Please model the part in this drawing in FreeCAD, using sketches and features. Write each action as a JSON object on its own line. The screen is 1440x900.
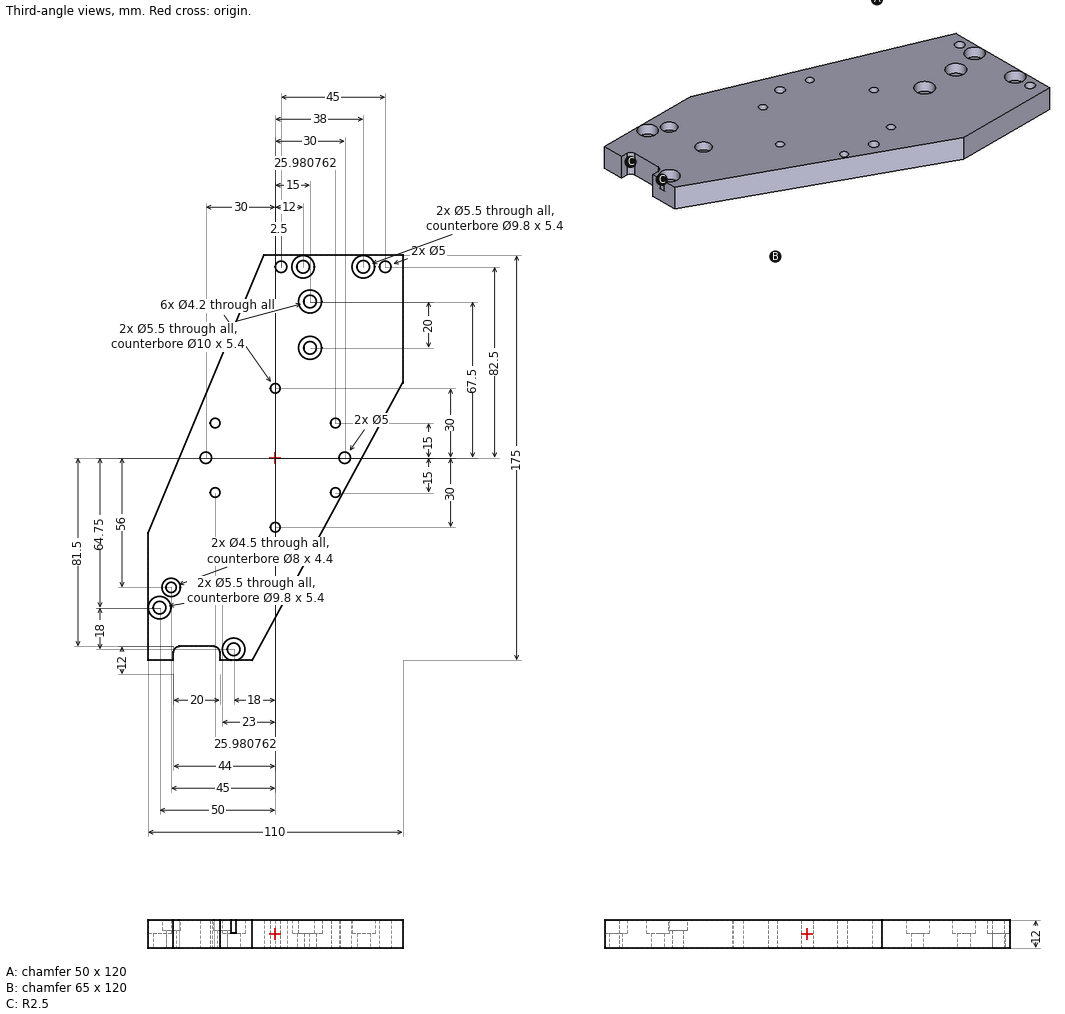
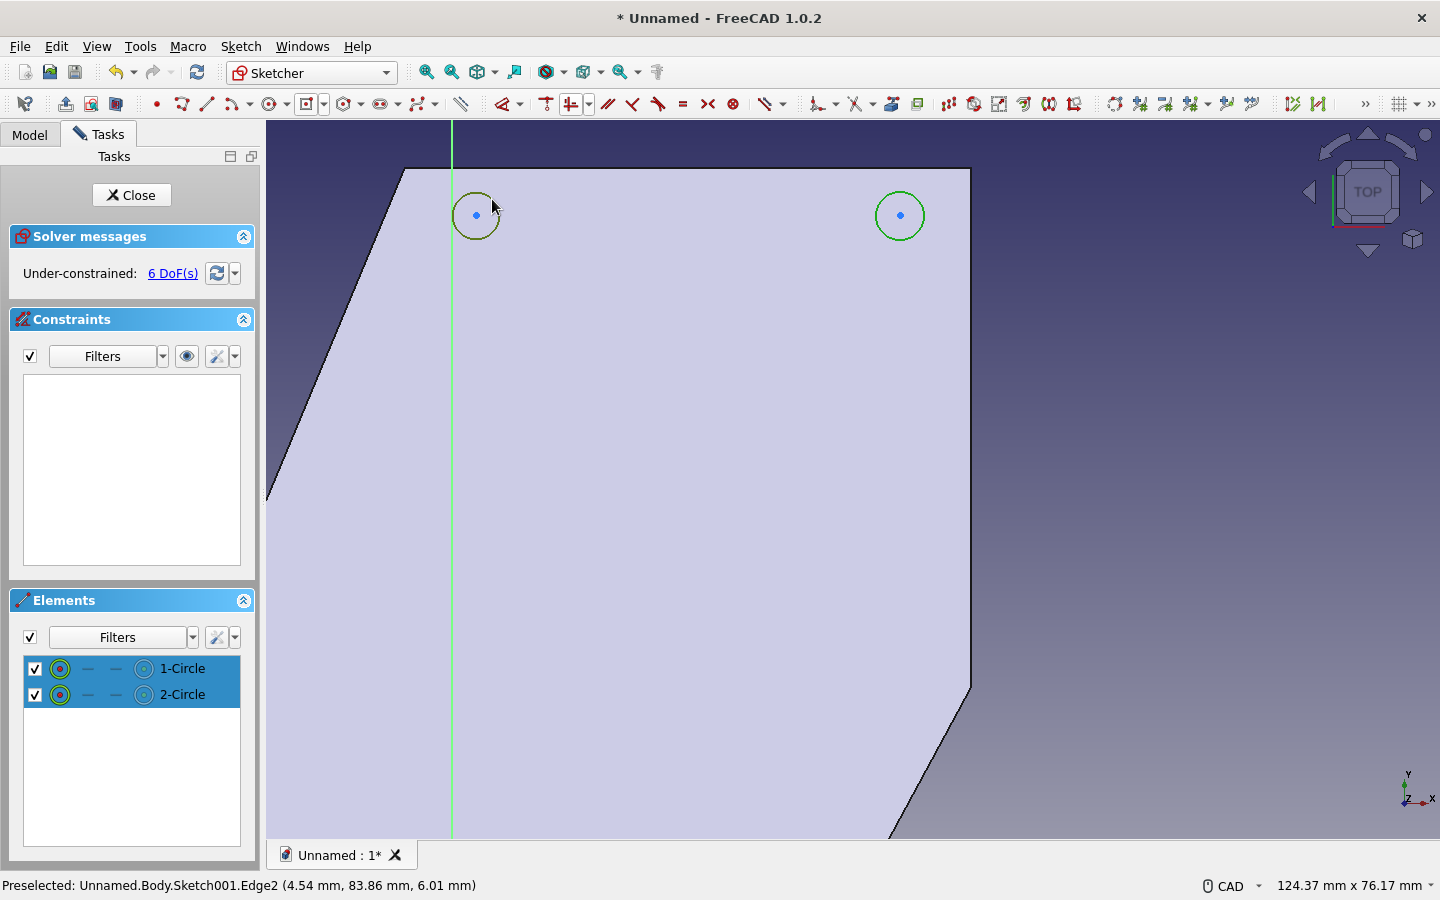
{"action": "key", "text": "e"}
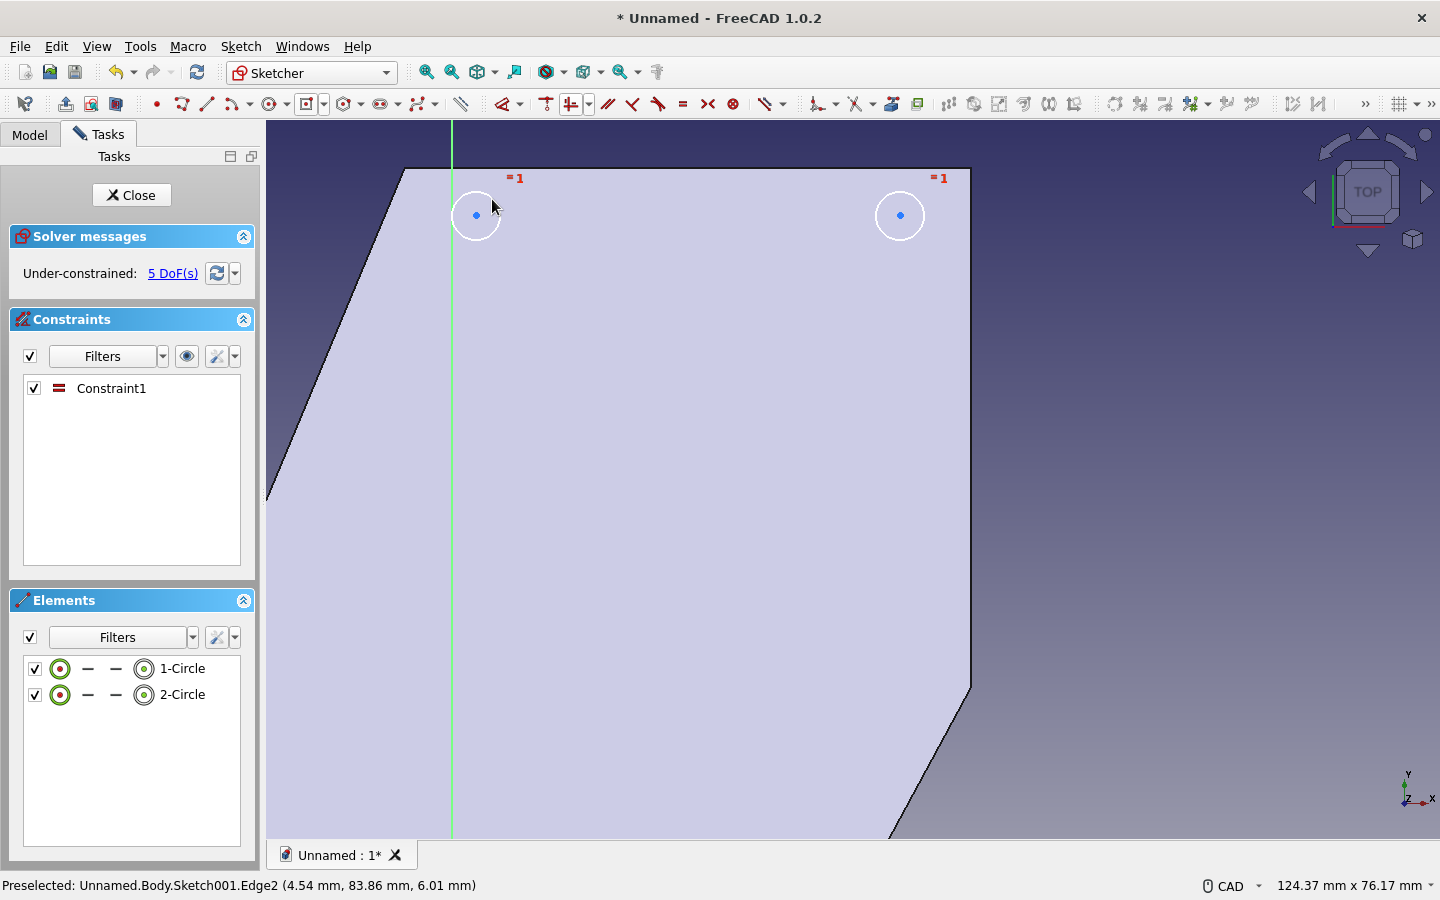
{"action": "left_click", "coordinate": [900, 216]}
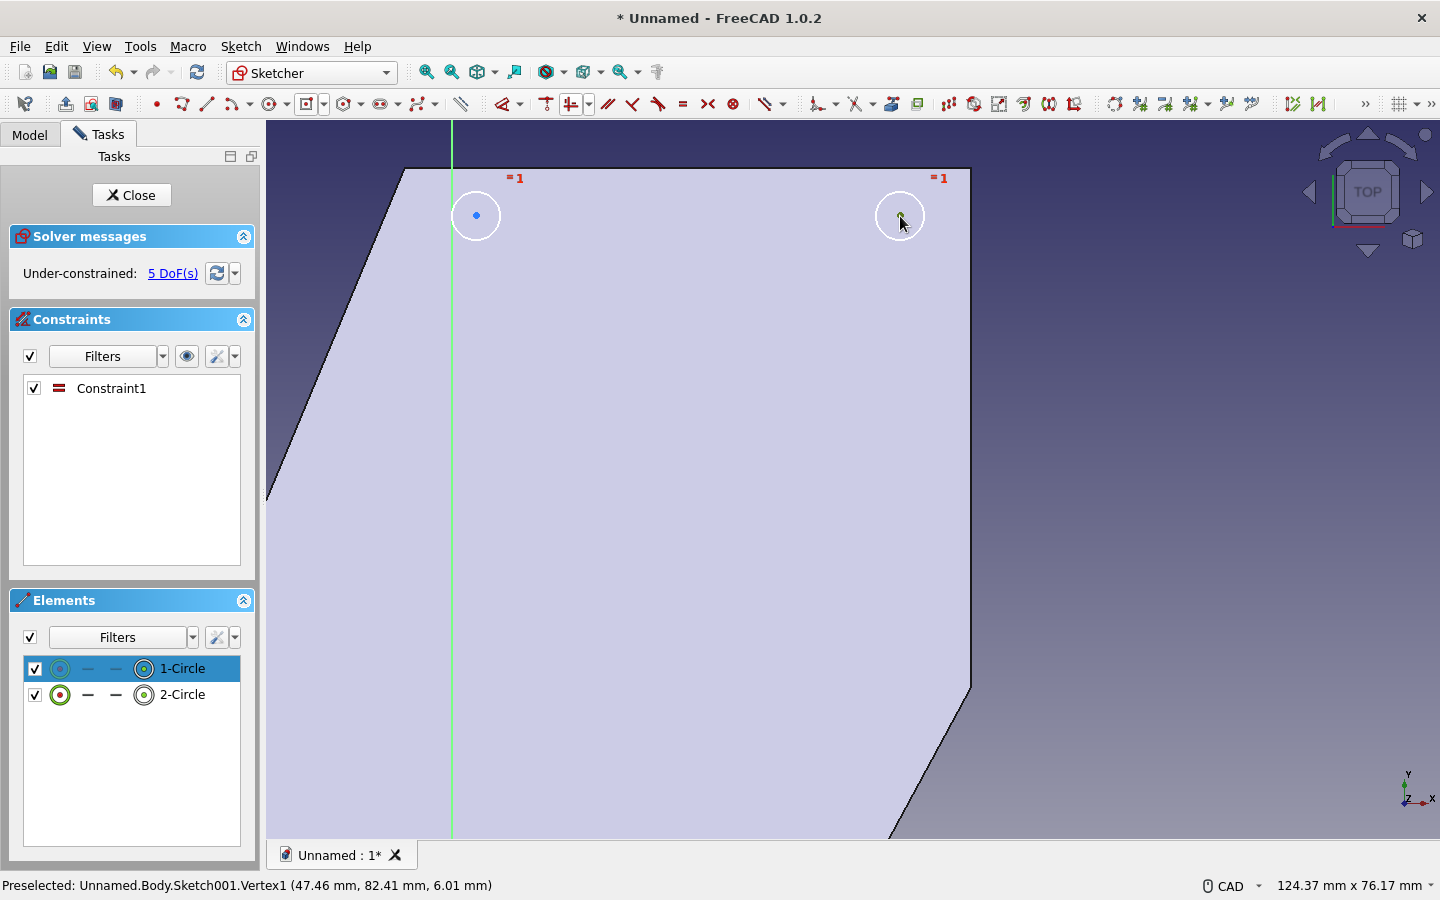
{"action": "left_click", "coordinate": [476, 216]}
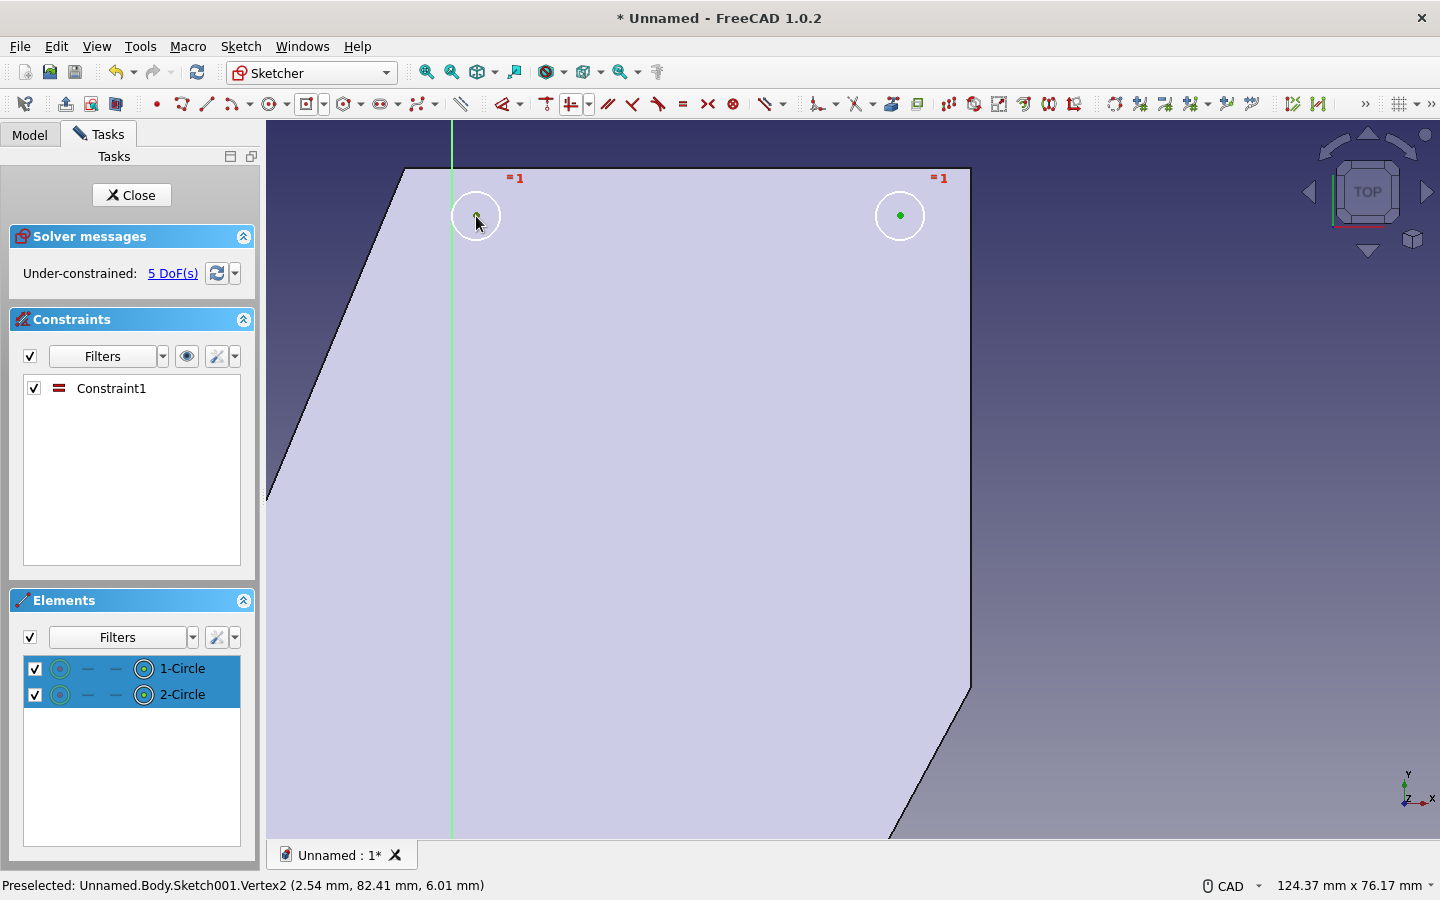
{"action": "key", "text": "h"}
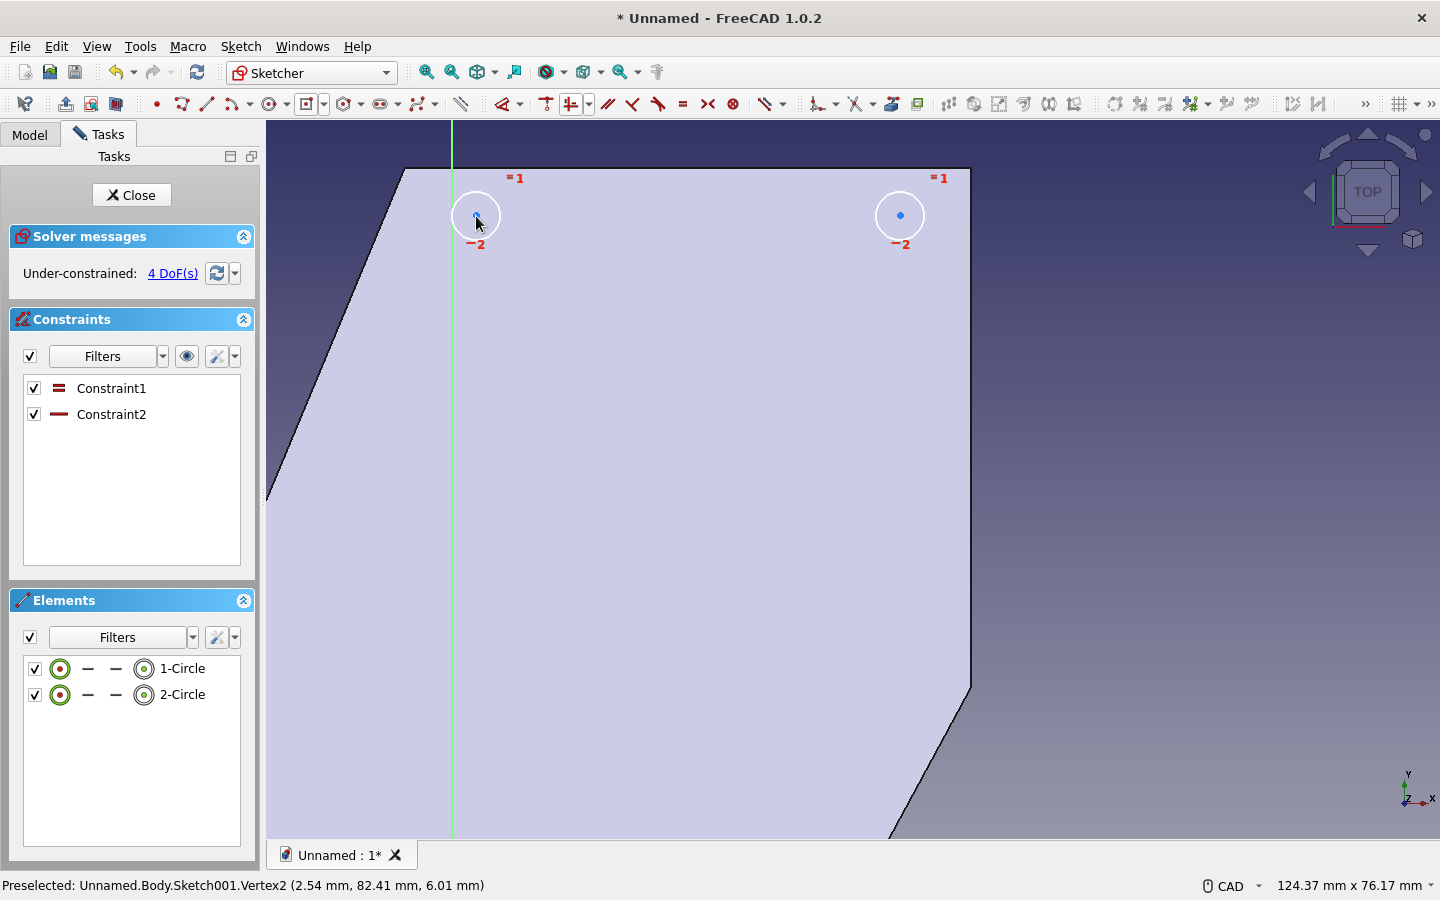
{"action": "left_click", "coordinate": [917, 199]}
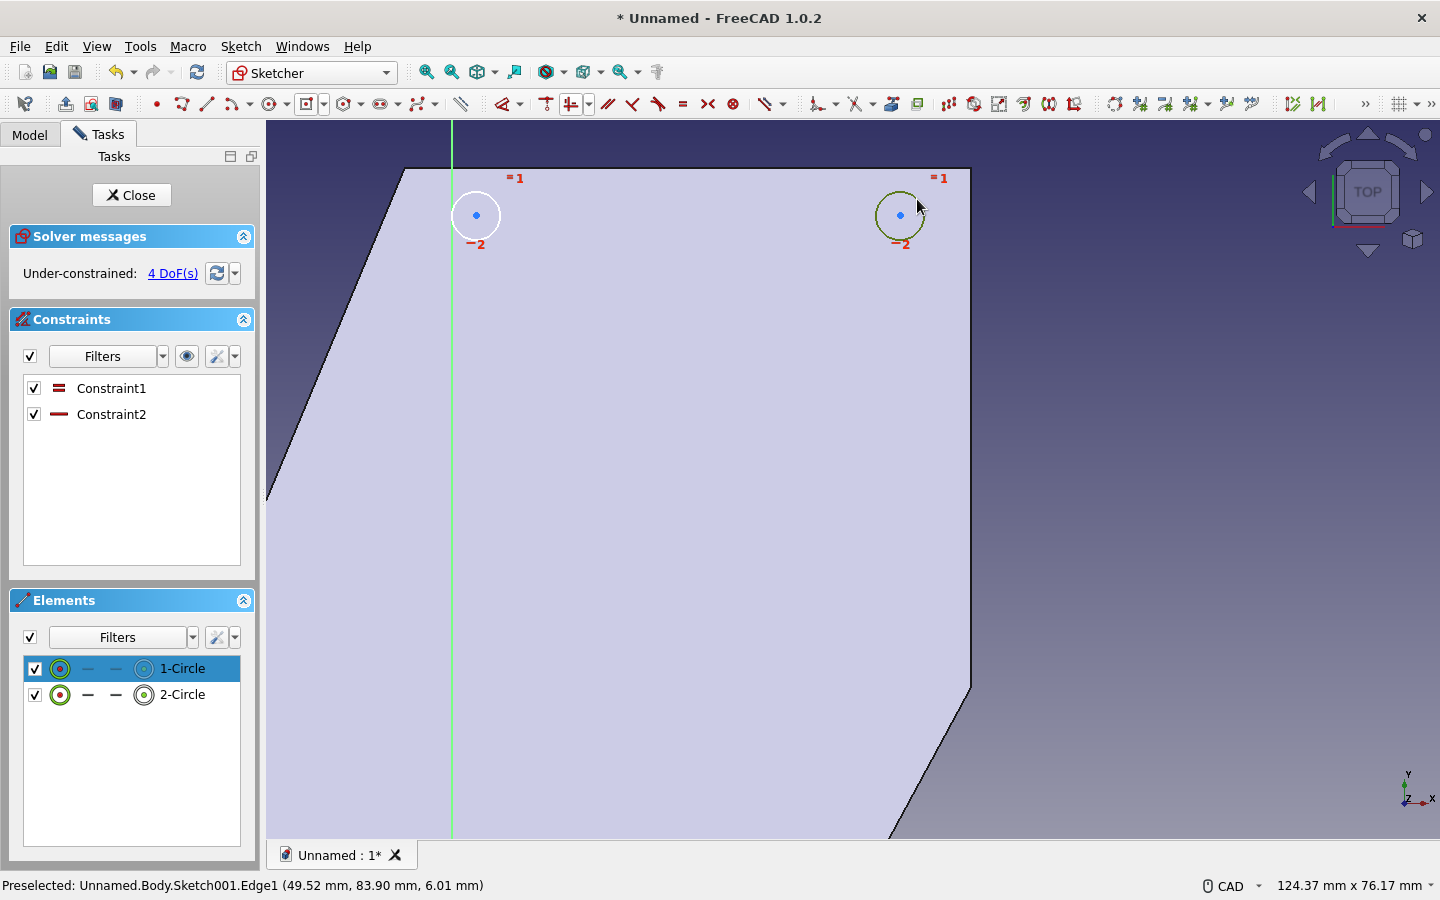
{"action": "key", "text": "k o"}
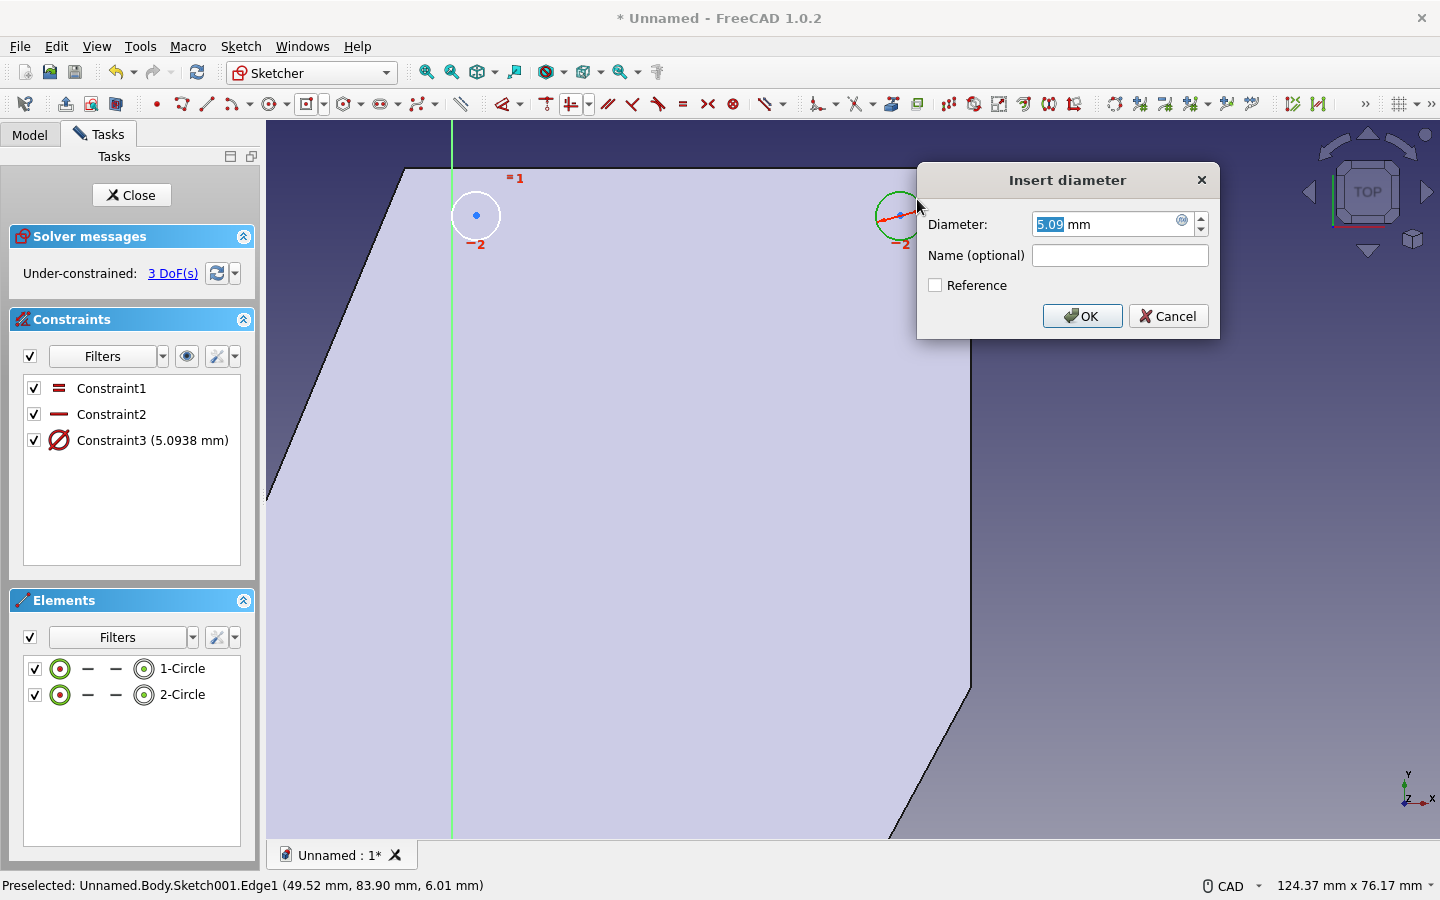
{"action": "type", "text": "5"}
{"action": "key", "text": "Return"}